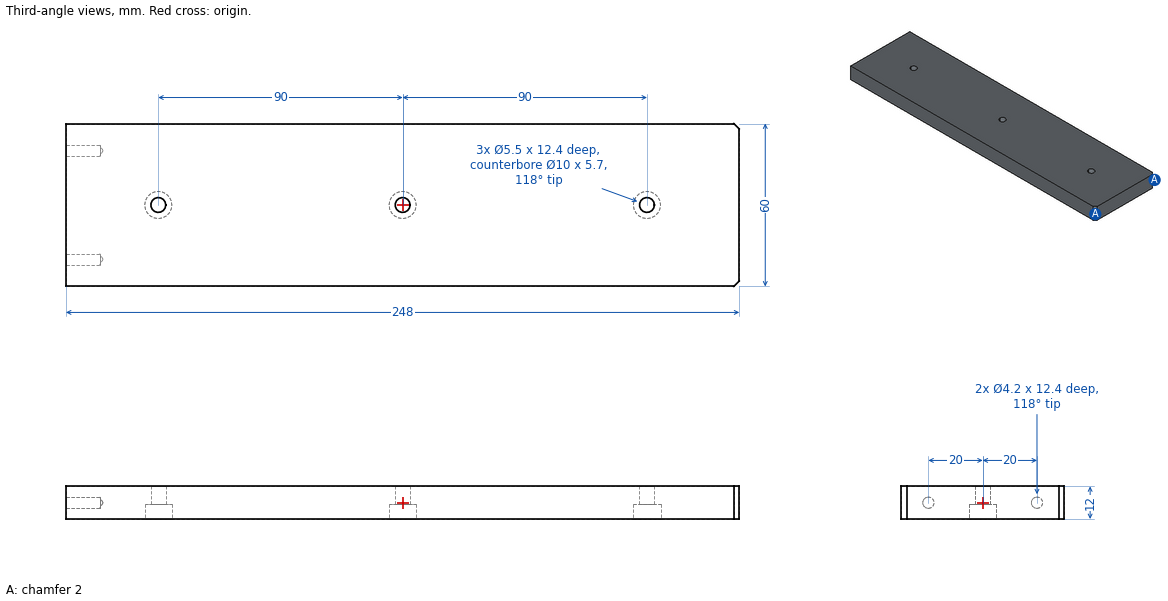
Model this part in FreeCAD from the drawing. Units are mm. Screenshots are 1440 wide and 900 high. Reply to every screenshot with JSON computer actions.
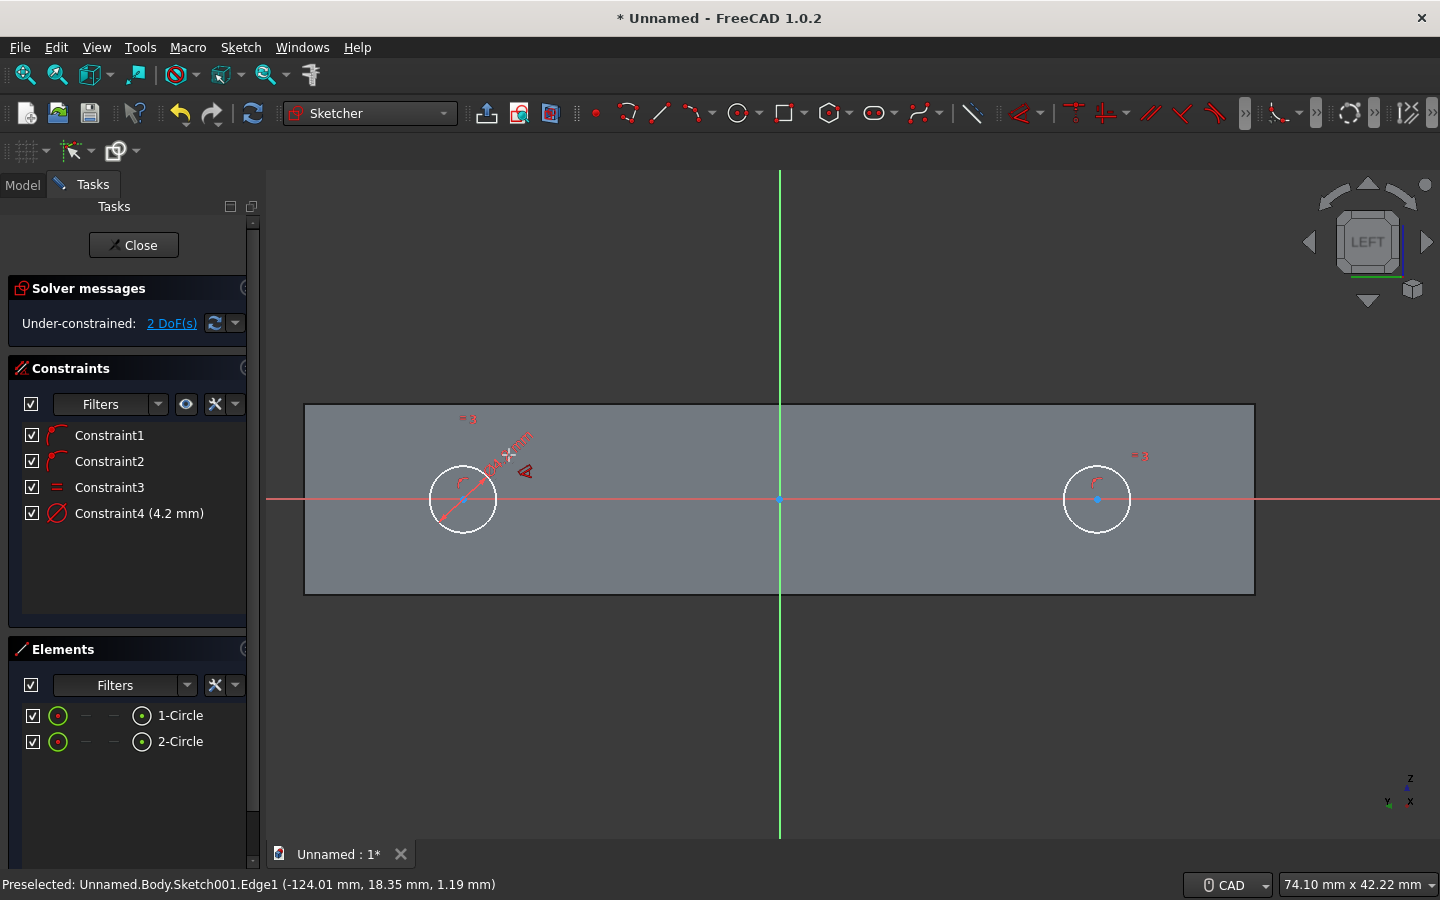
{"action": "left_click", "coordinate": [463, 499]}
{"action": "left_click", "coordinate": [621, 533]}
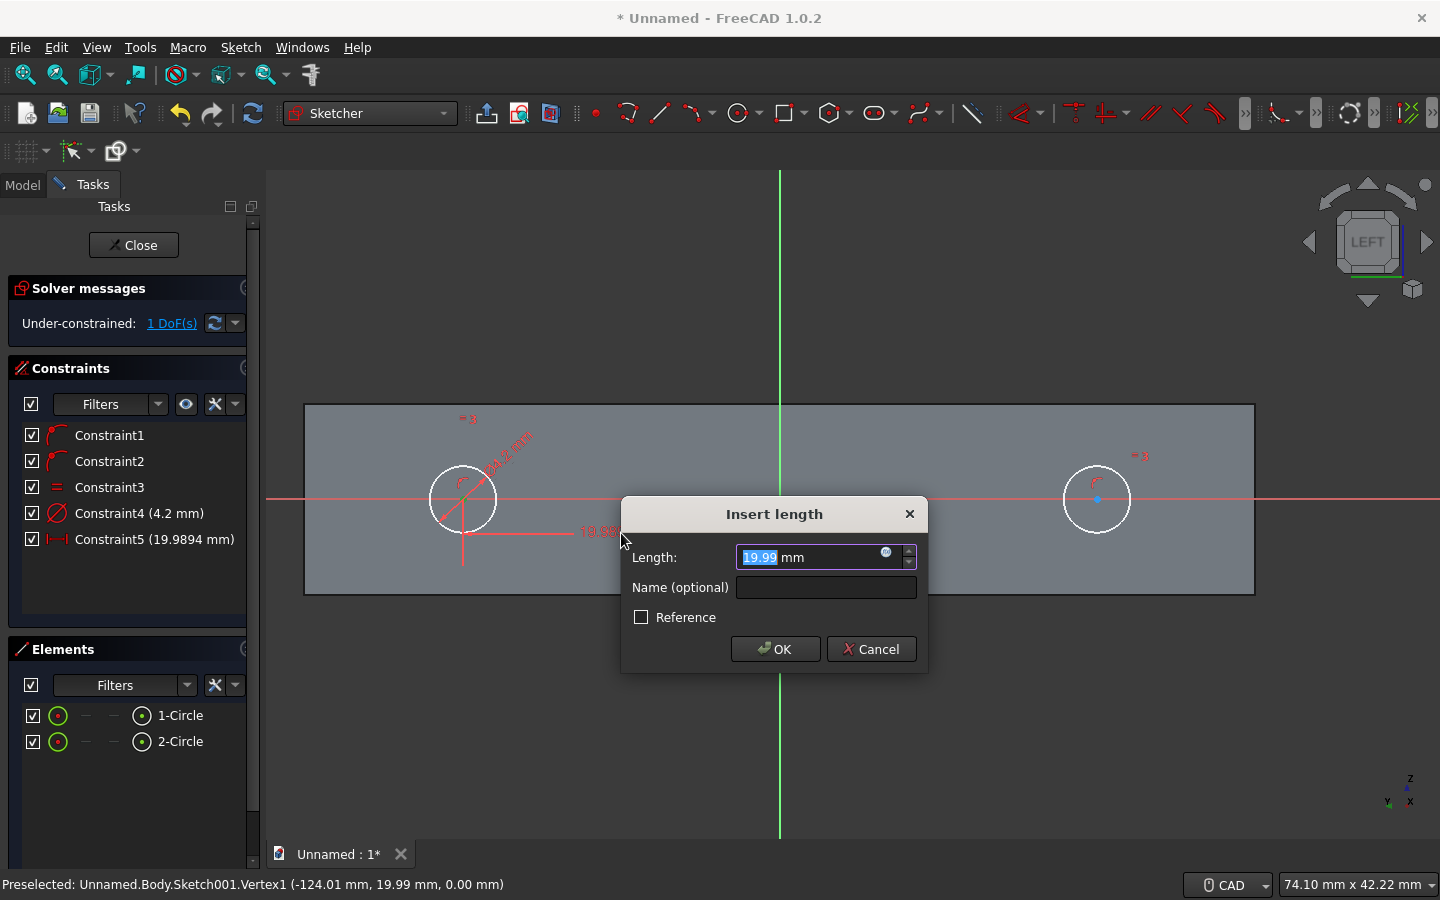
{"action": "type", "text": "20"}
{"action": "key", "text": "Return"}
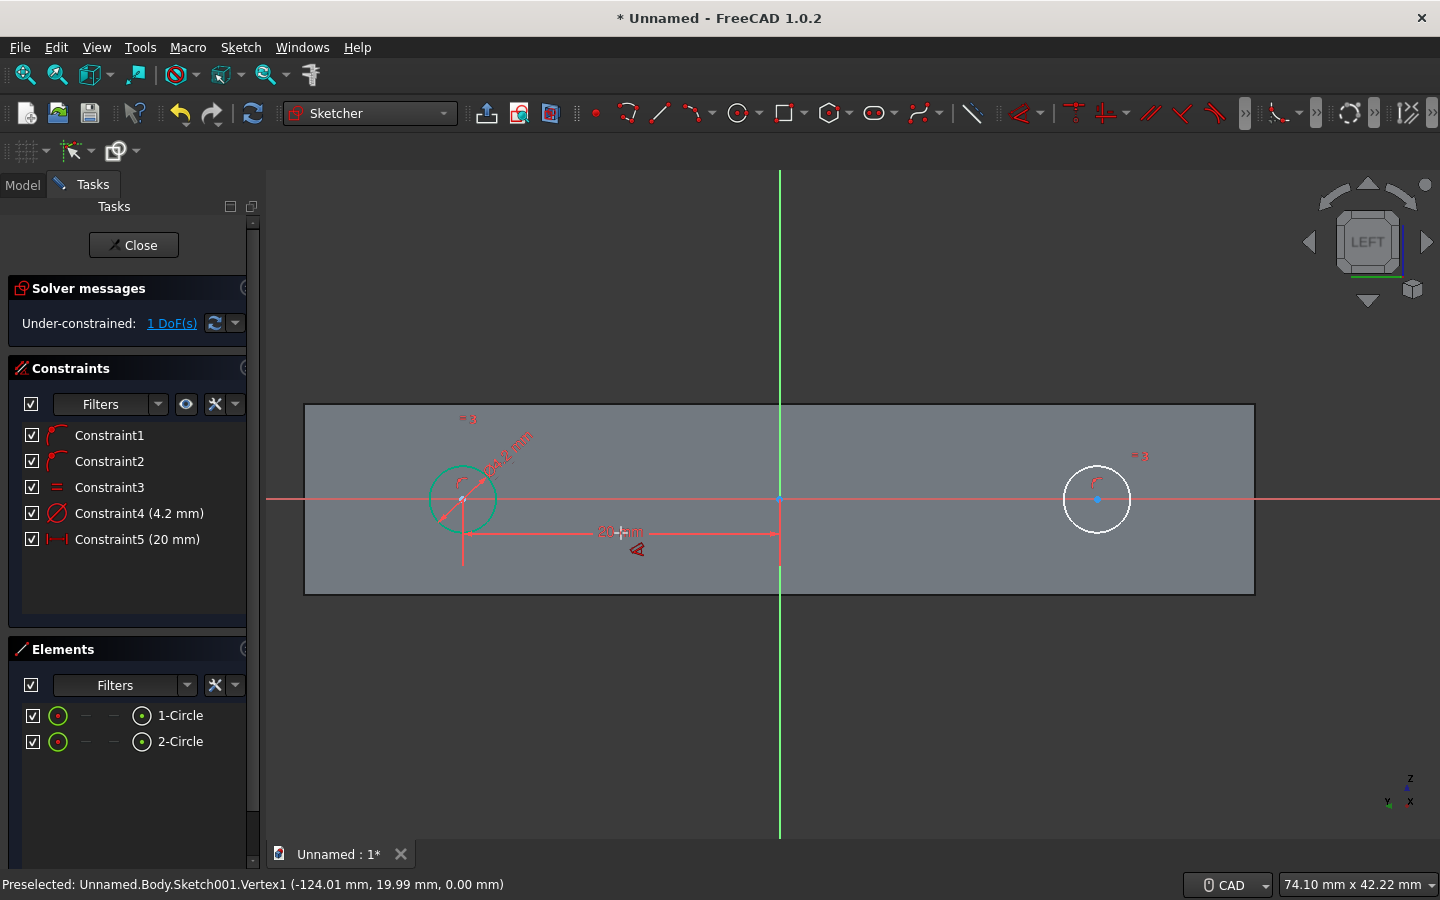
{"action": "left_click", "coordinate": [1097, 499]}
{"action": "left_click", "coordinate": [938, 533]}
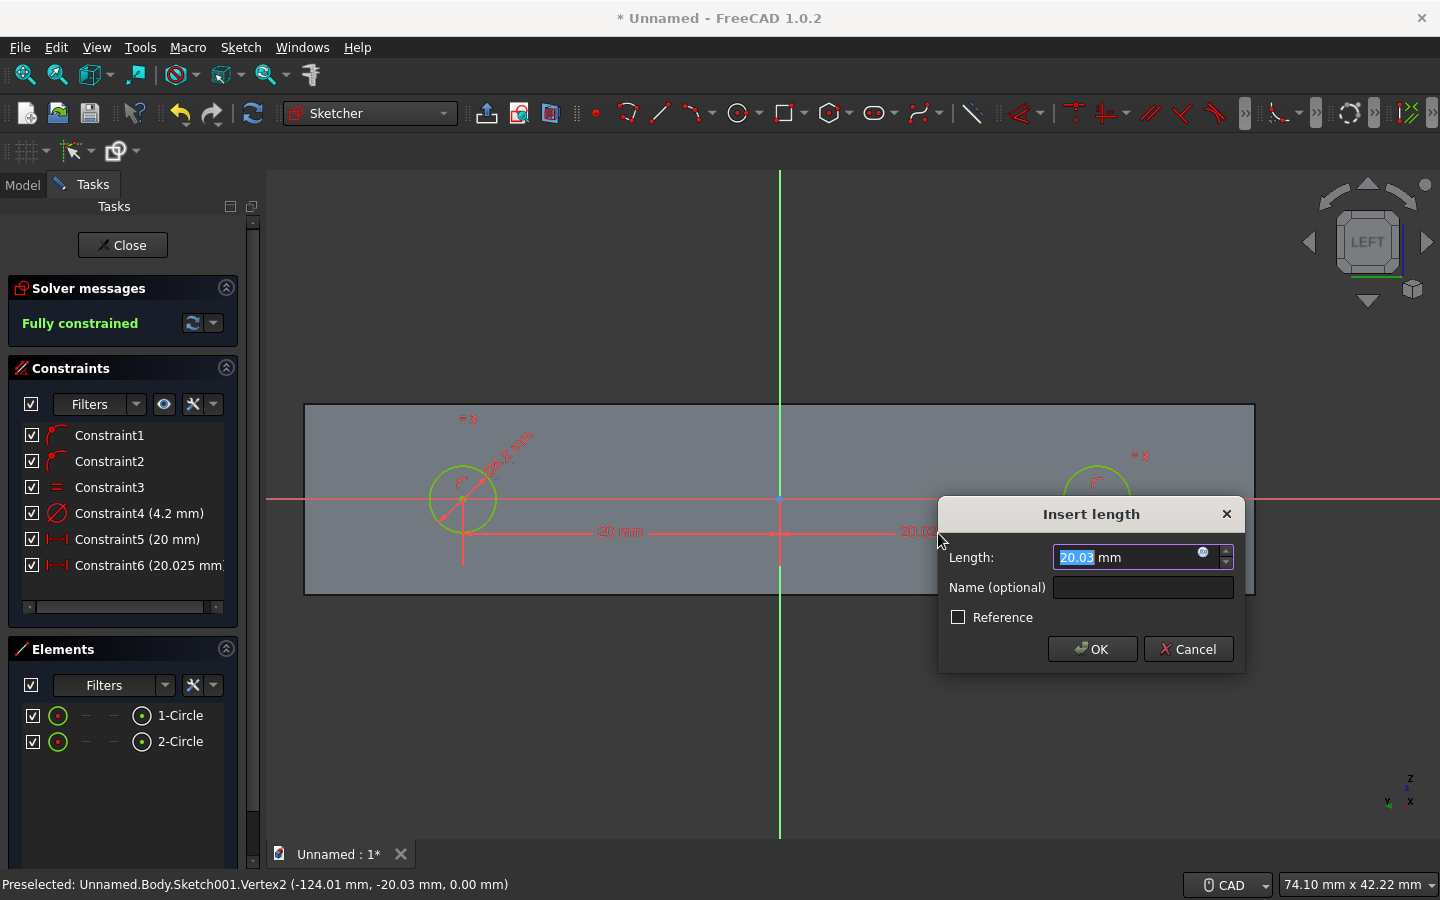
{"action": "type", "text": "20"}
{"action": "key", "text": "Return"}
{"action": "key", "text": "Escape"}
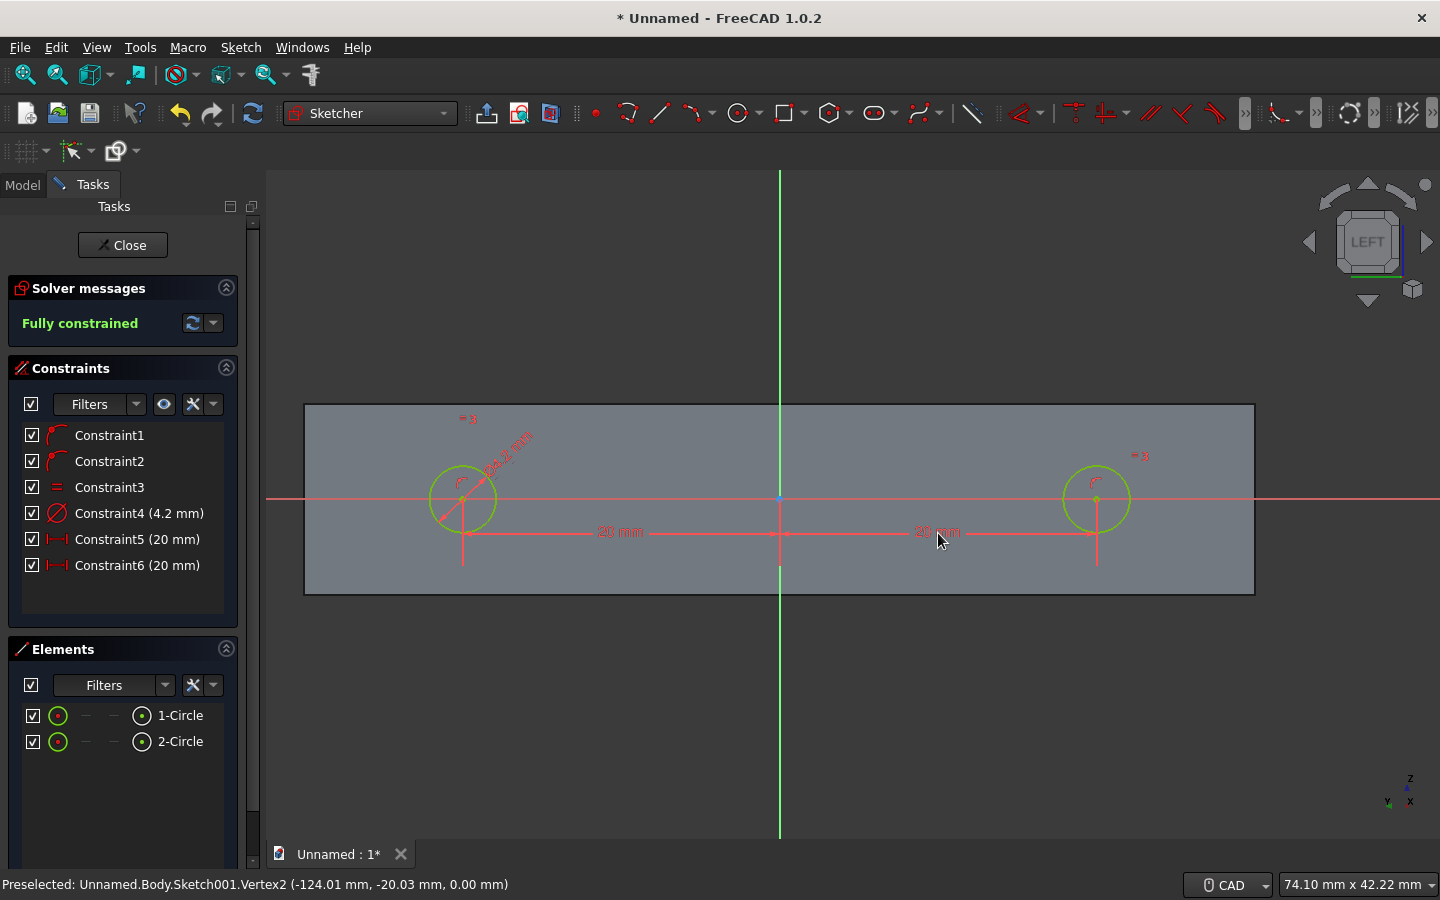
{"action": "left_click", "coordinate": [123, 245]}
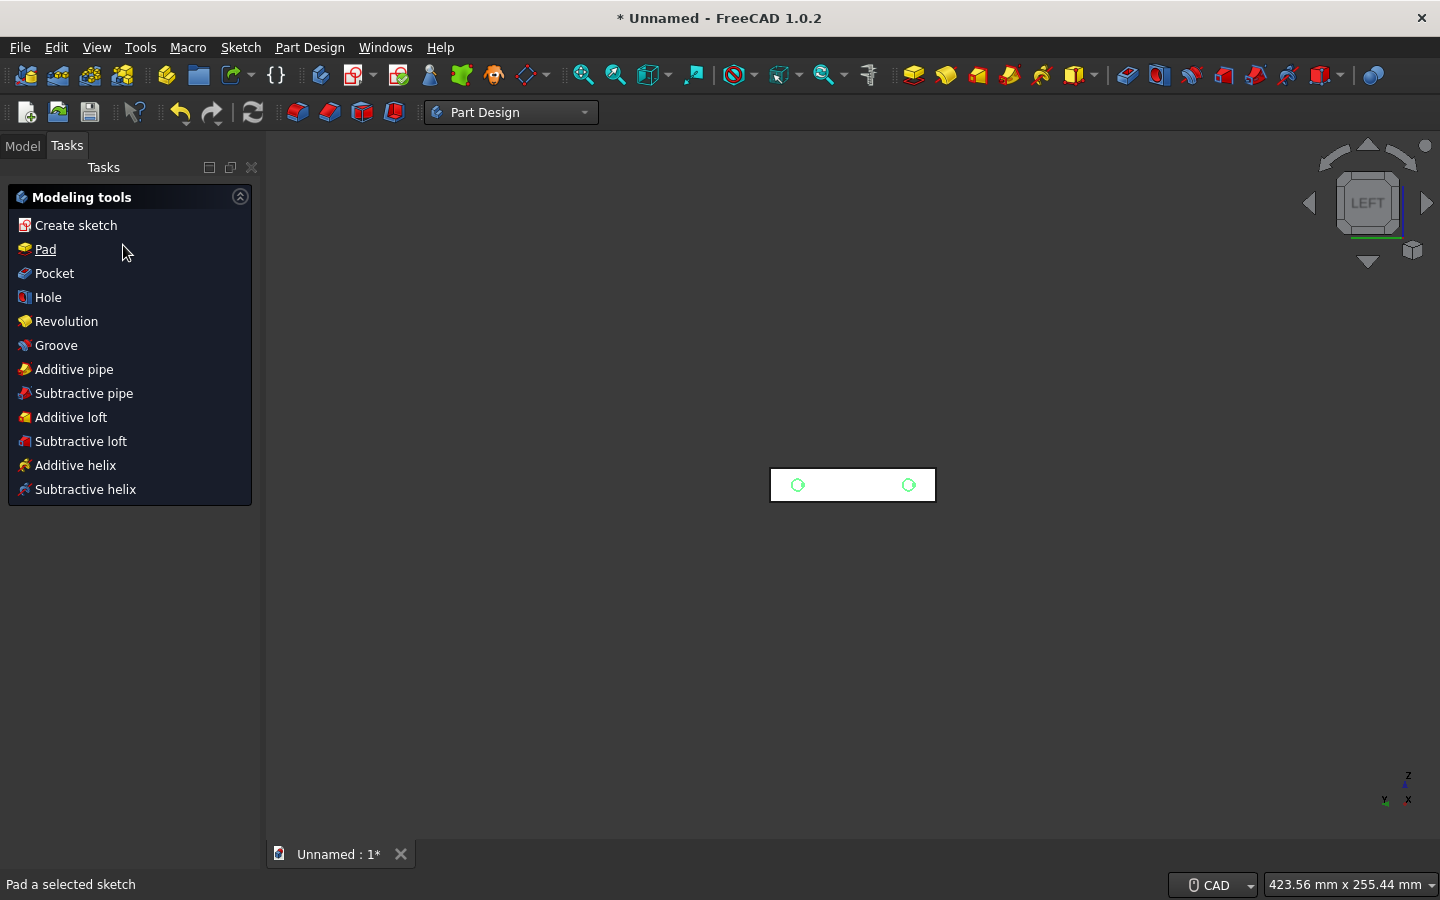
{"action": "left_click", "coordinate": [1160, 76]}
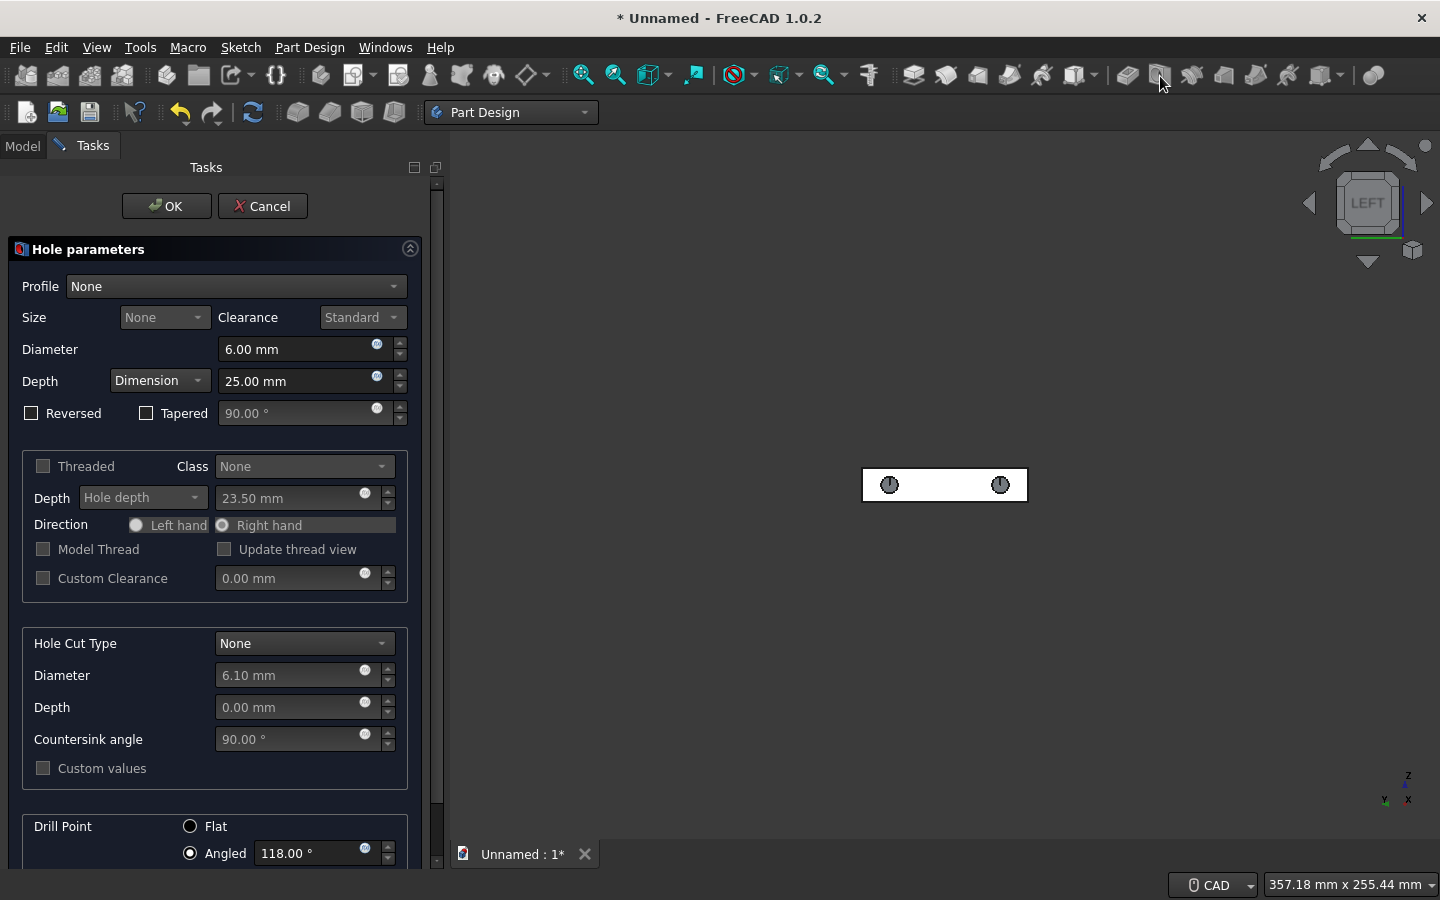
{"action": "triple_click", "coordinate": [305, 349]}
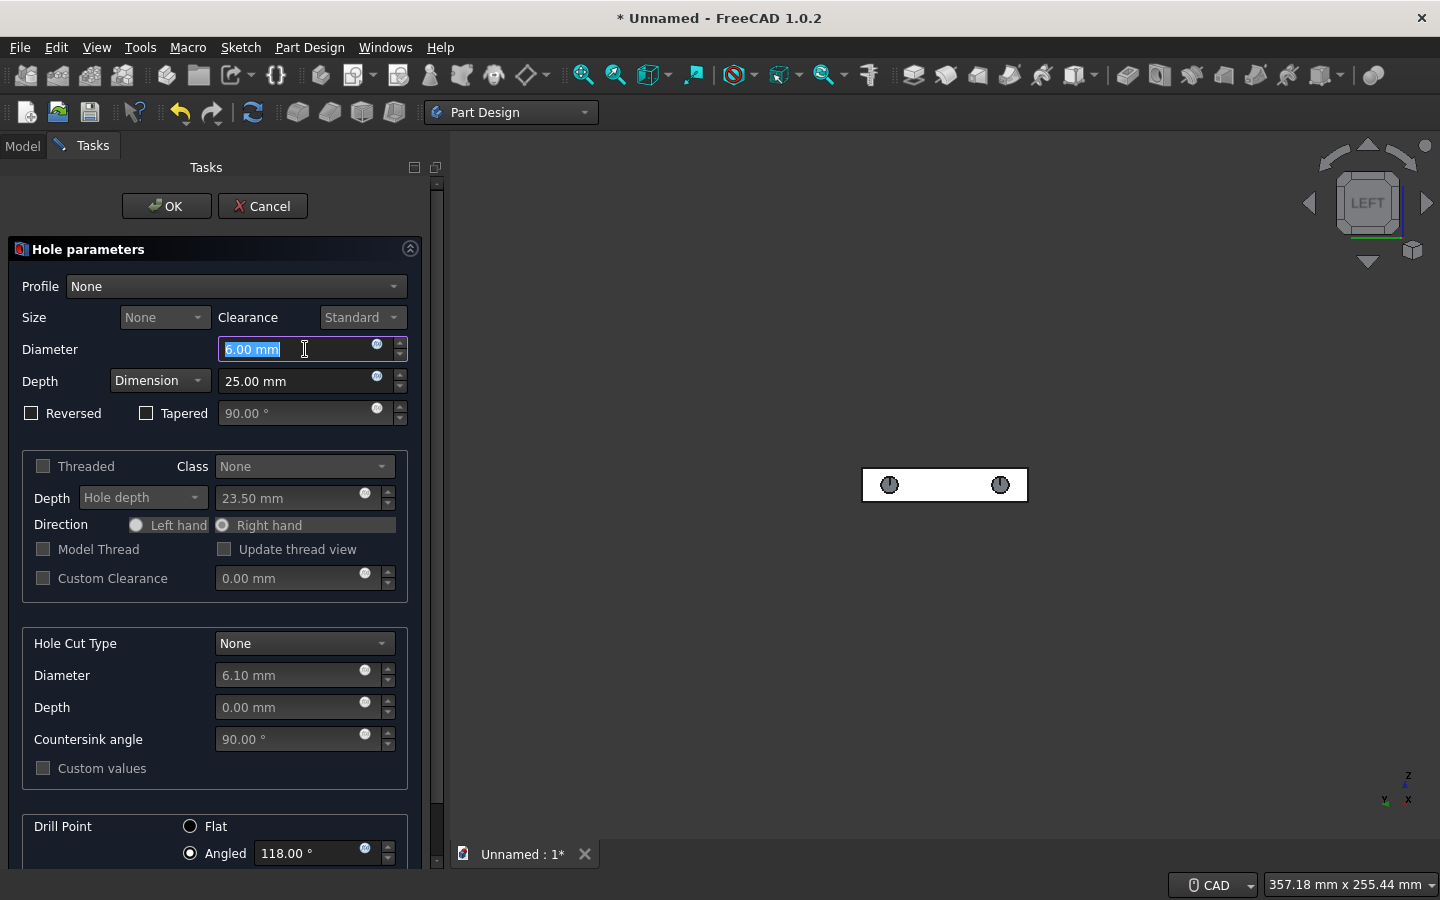
{"action": "type", "text": "4.2"}
{"action": "key", "text": "Tab"}